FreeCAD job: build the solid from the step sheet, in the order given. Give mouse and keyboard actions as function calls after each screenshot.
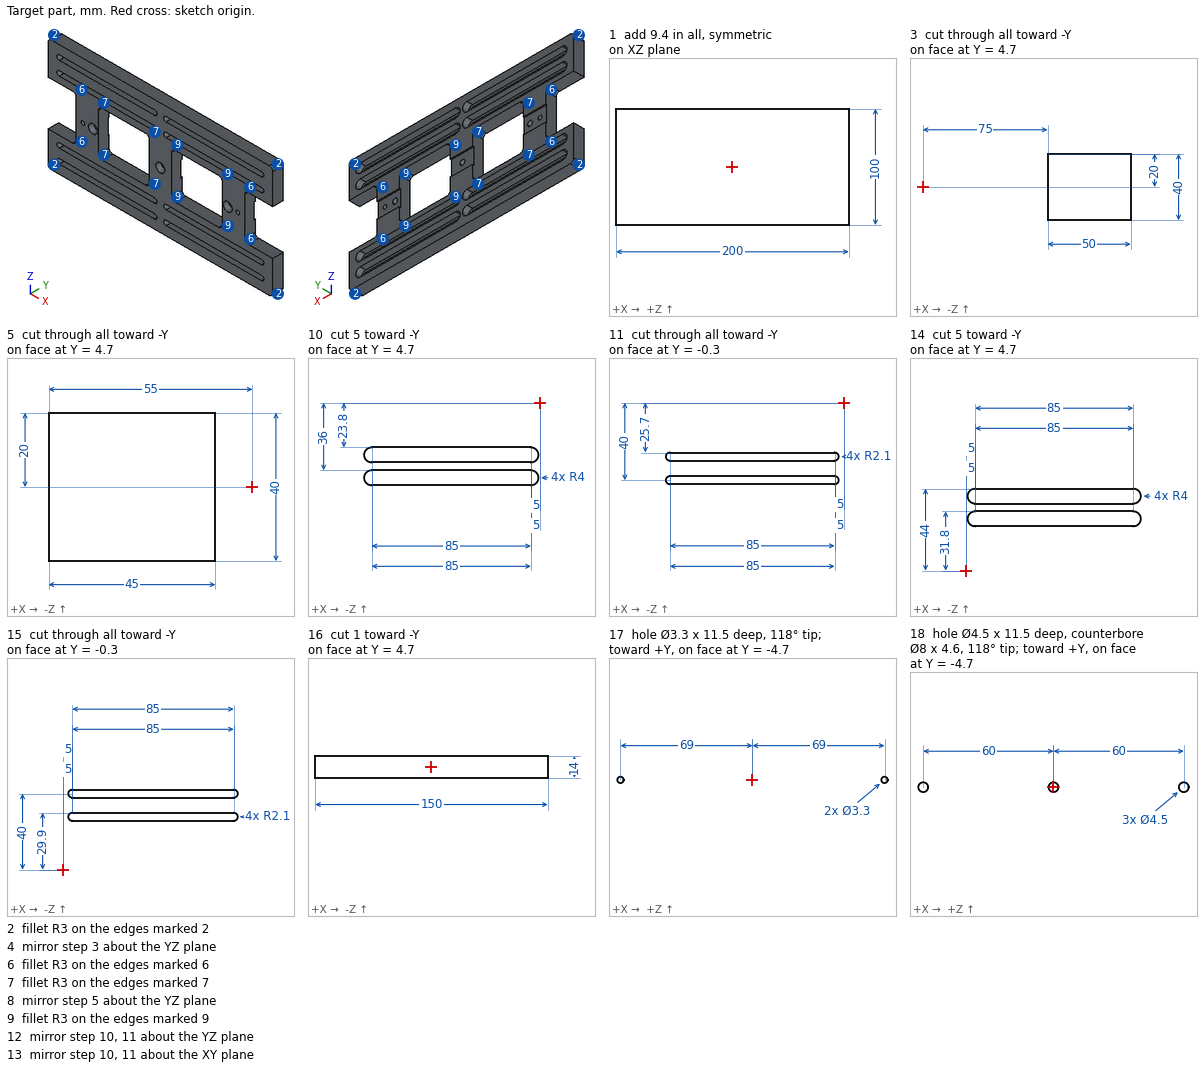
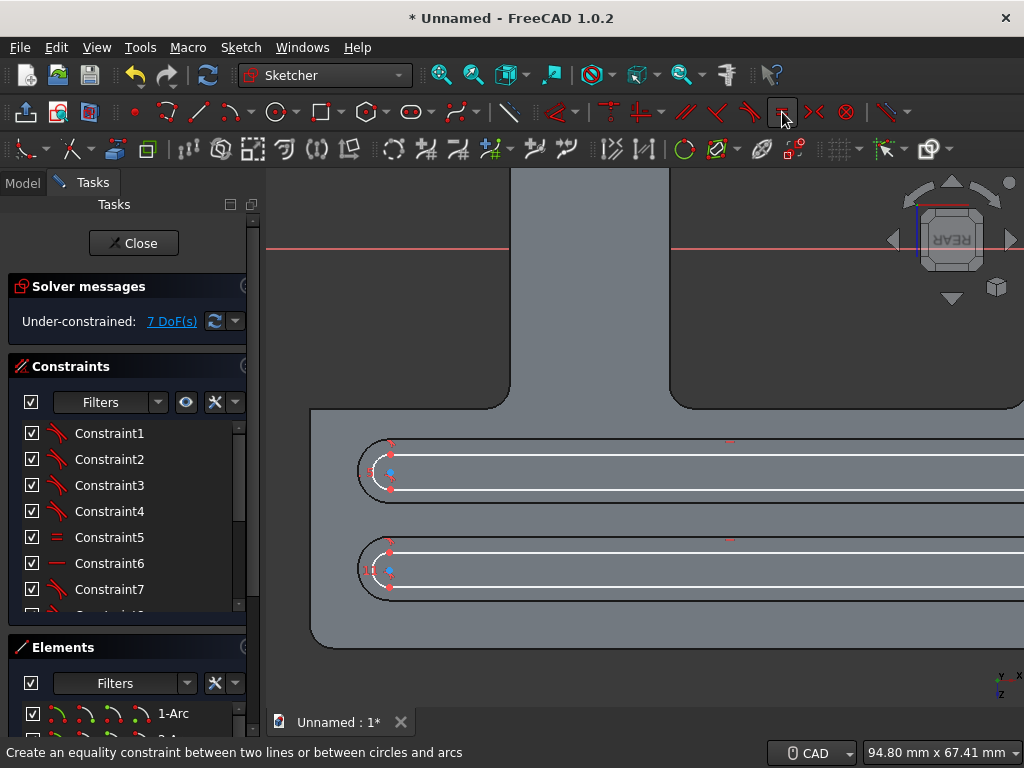
key(d)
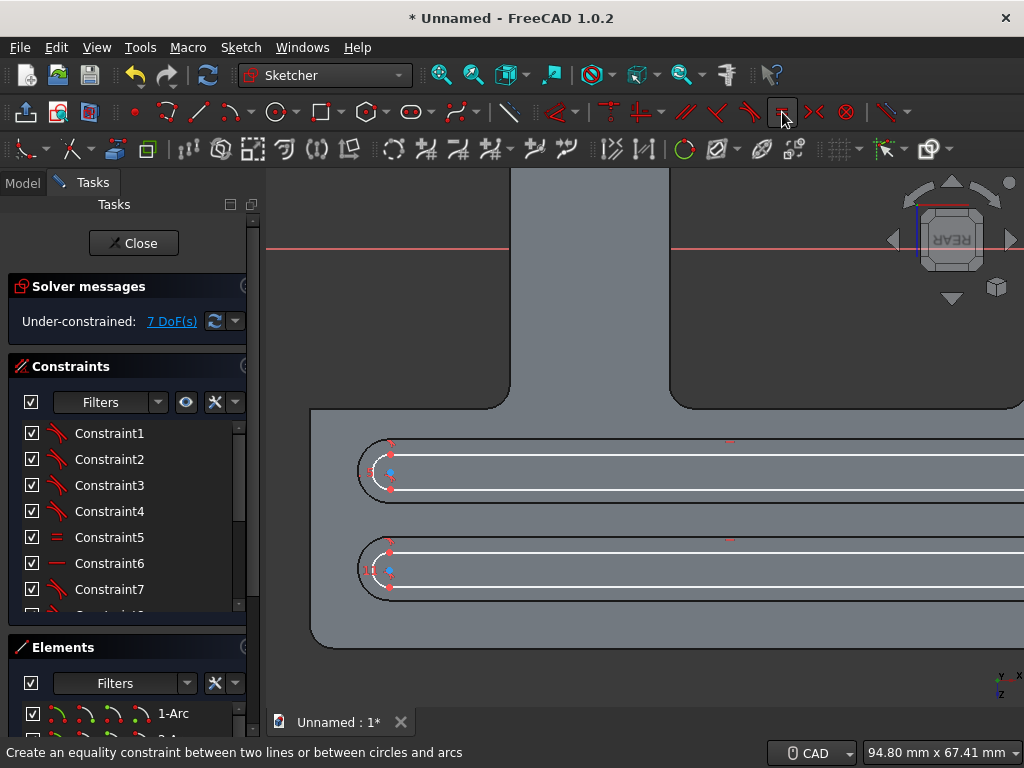
scroll(376, 462, up, 5)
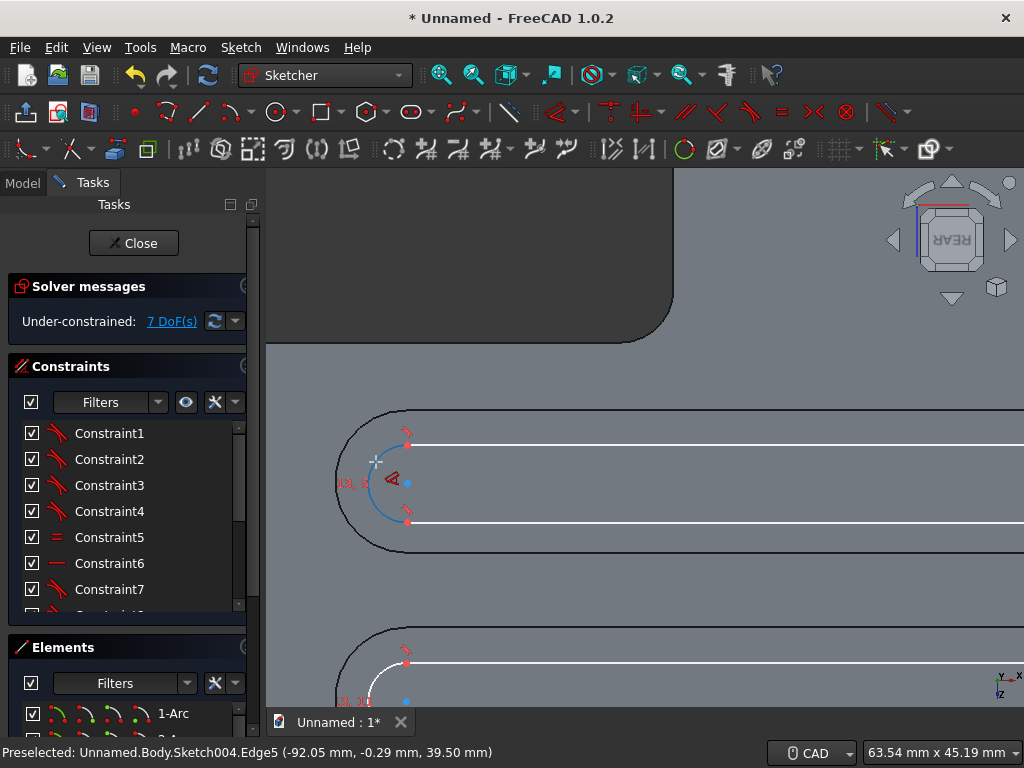
click(376, 461)
click(350, 442)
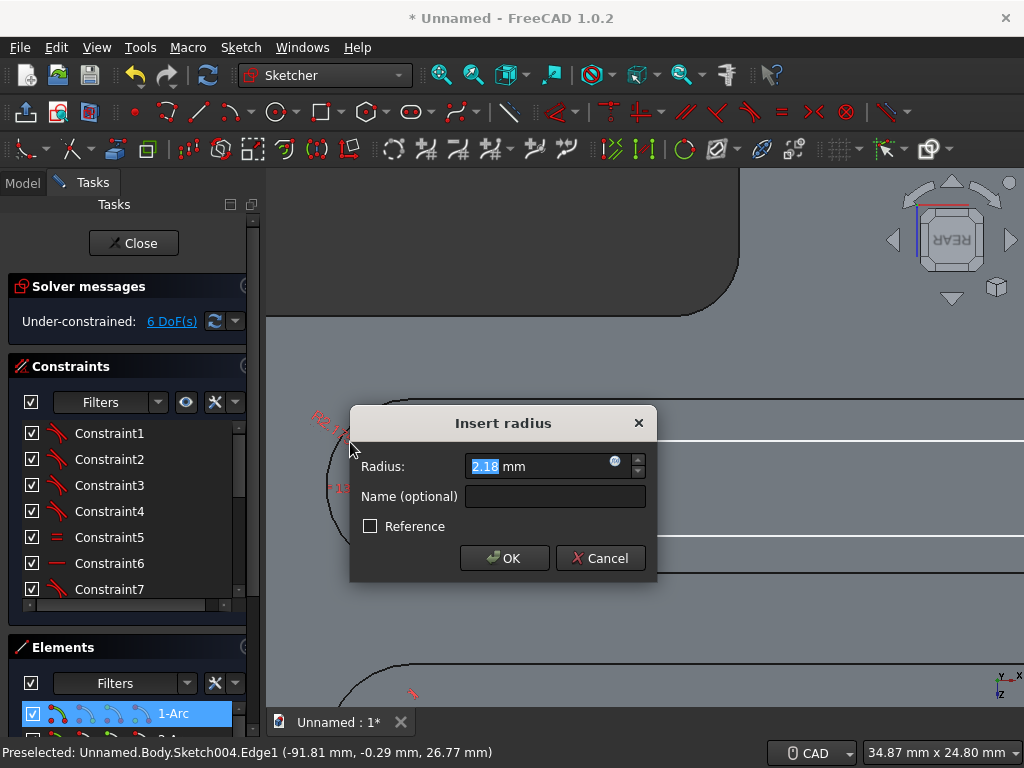
text(2.1)
key(Return)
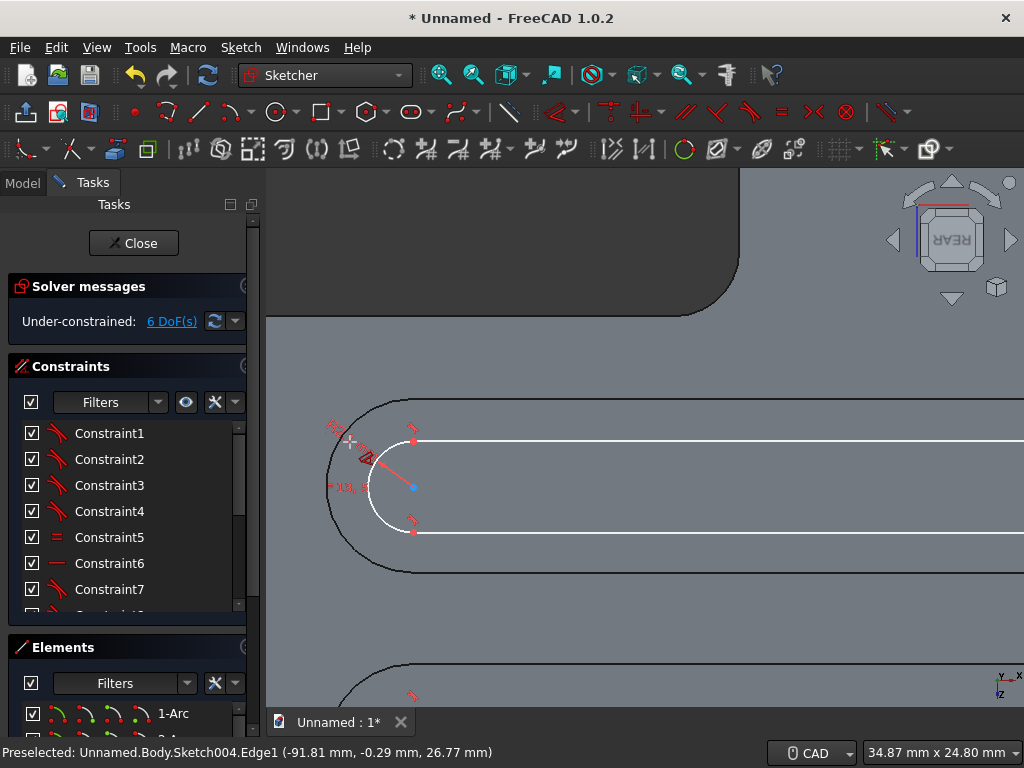
scroll(376, 462, down, 8)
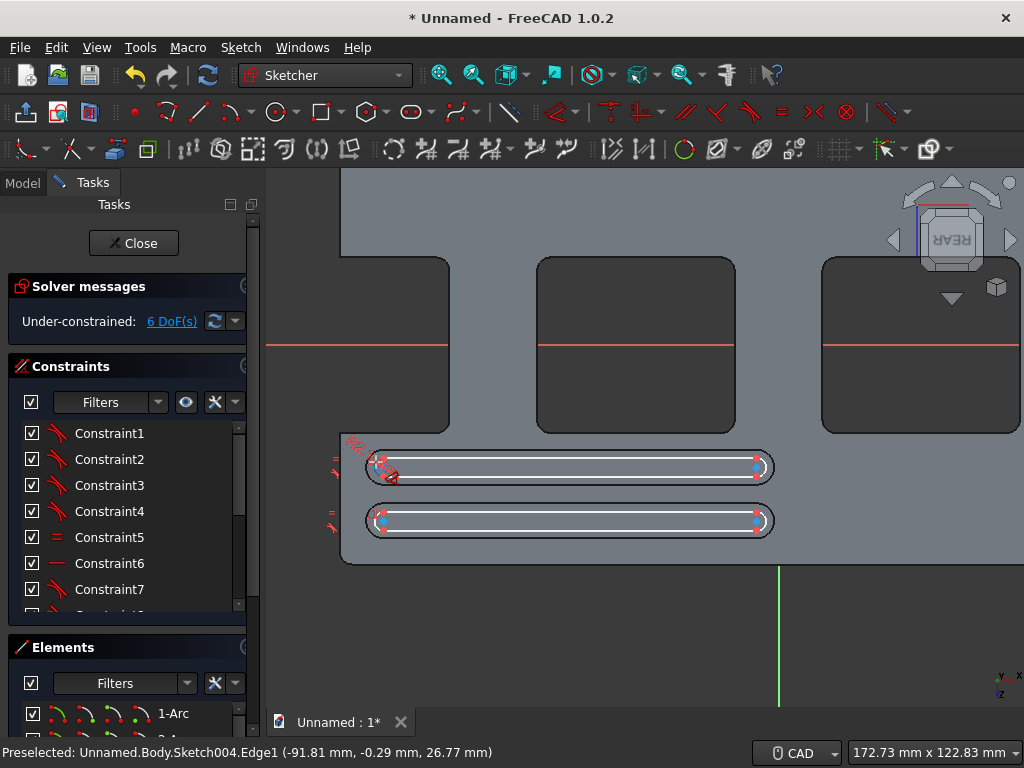
click(458, 458)
click(570, 492)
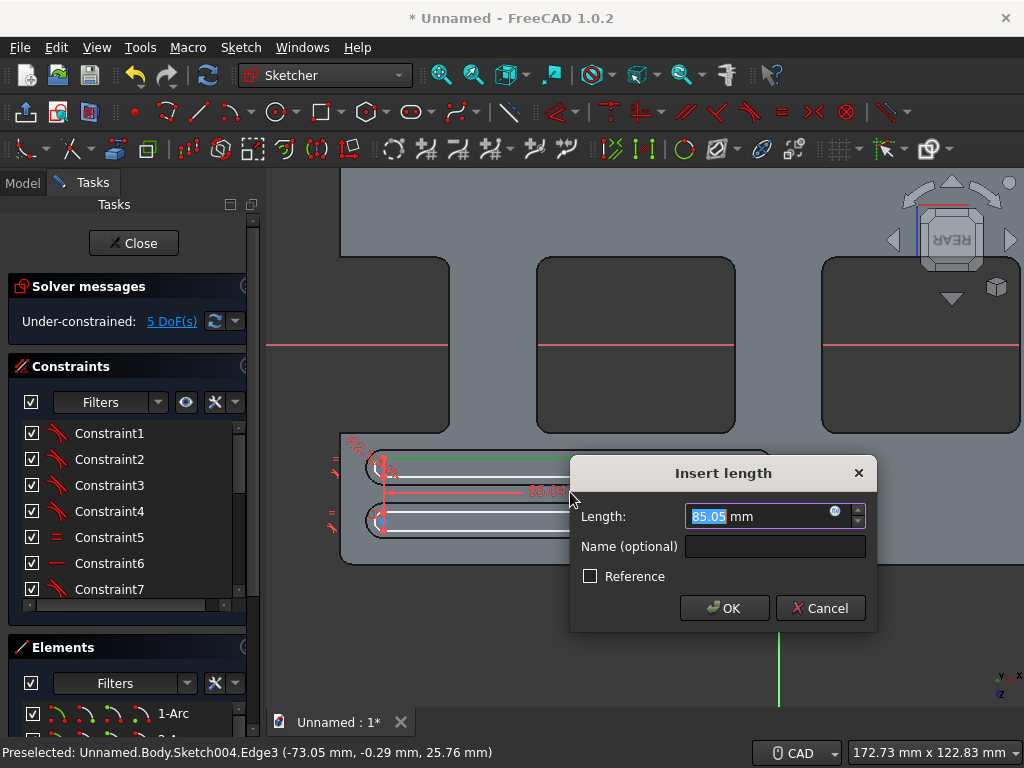
text(85)
key(Return)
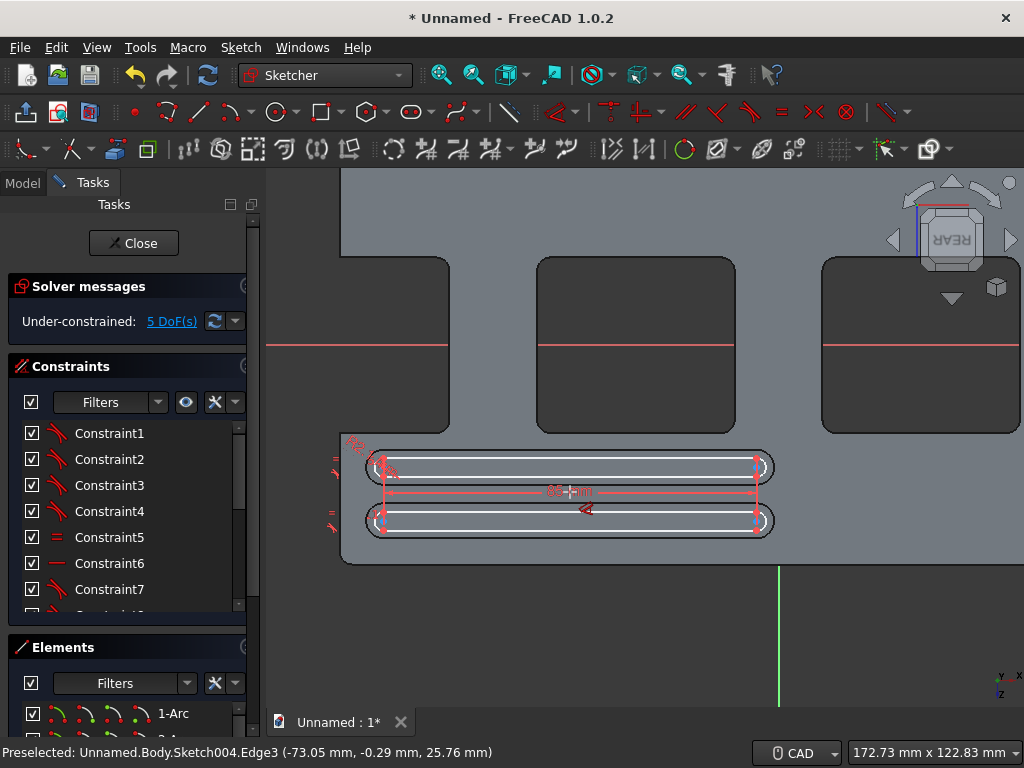
click(496, 512)
click(570, 546)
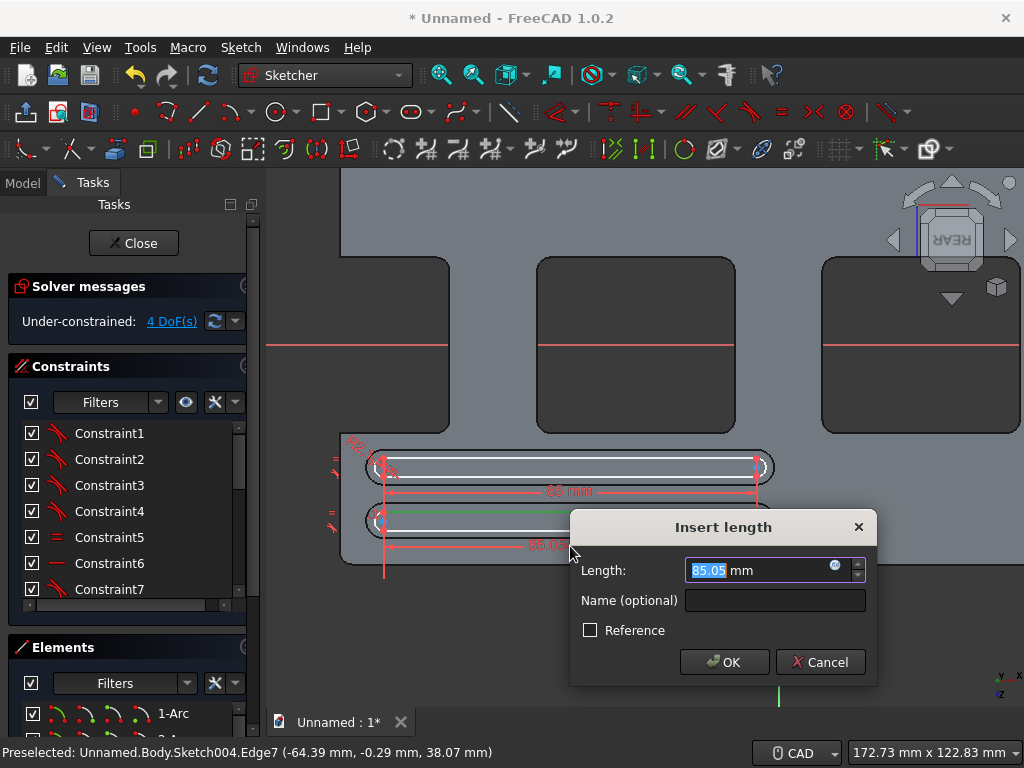
text(85)
key(Return)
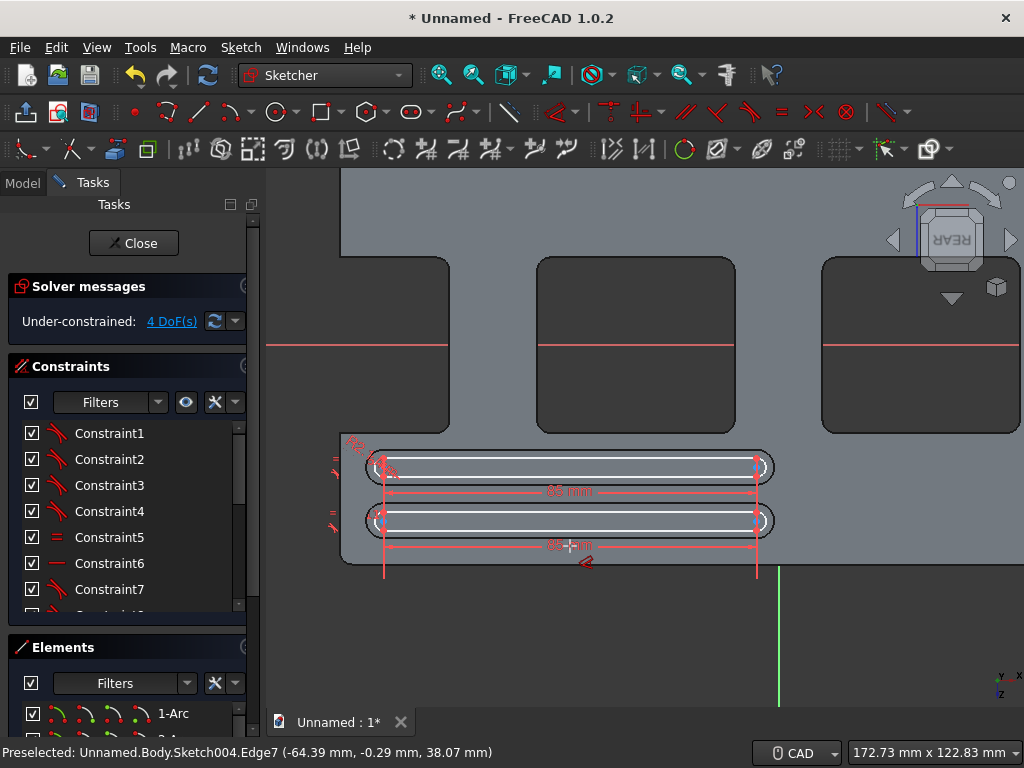
scroll(757, 477, up, 3)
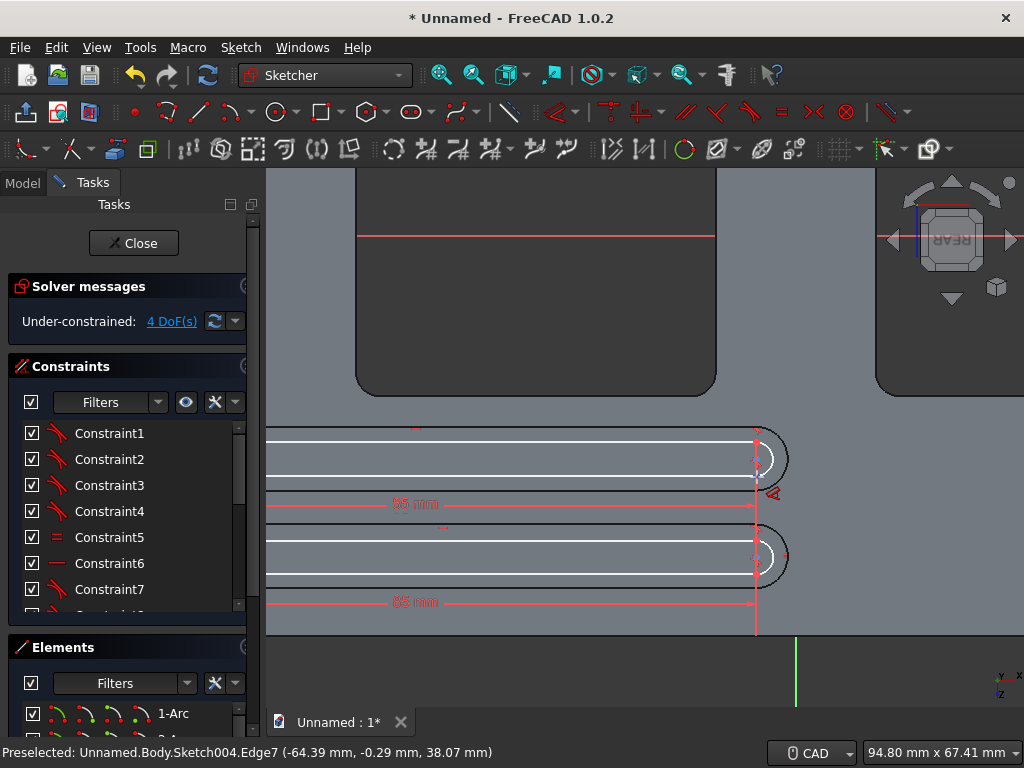
click(756, 476)
click(776, 202)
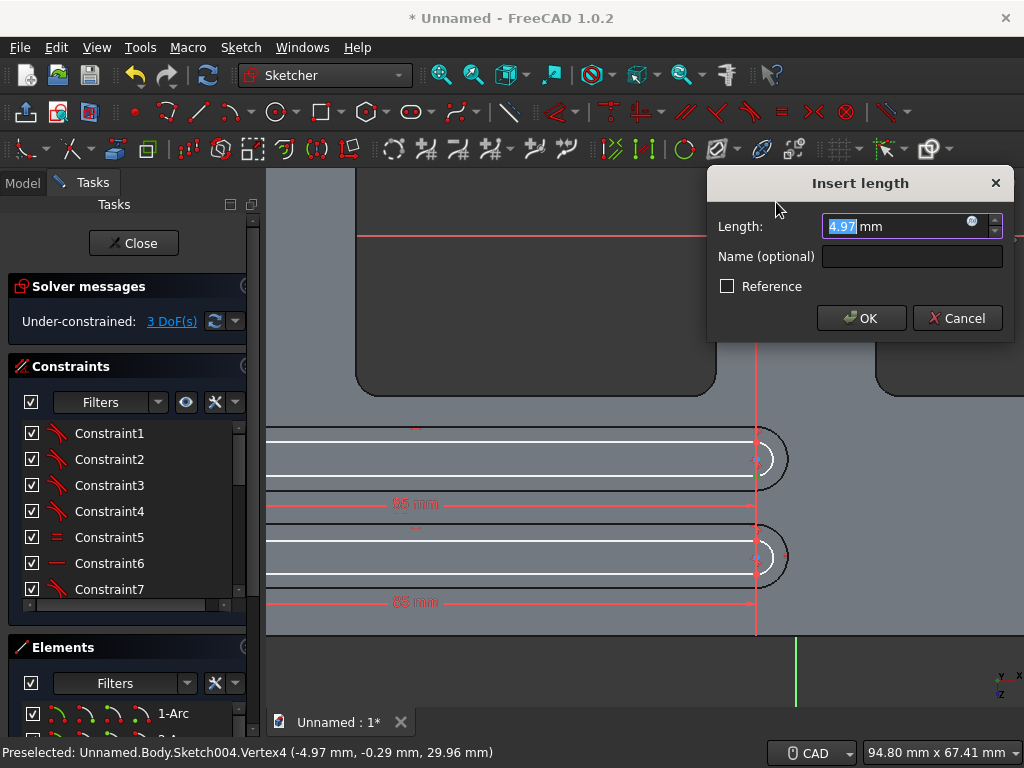
text(5)
key(Return)